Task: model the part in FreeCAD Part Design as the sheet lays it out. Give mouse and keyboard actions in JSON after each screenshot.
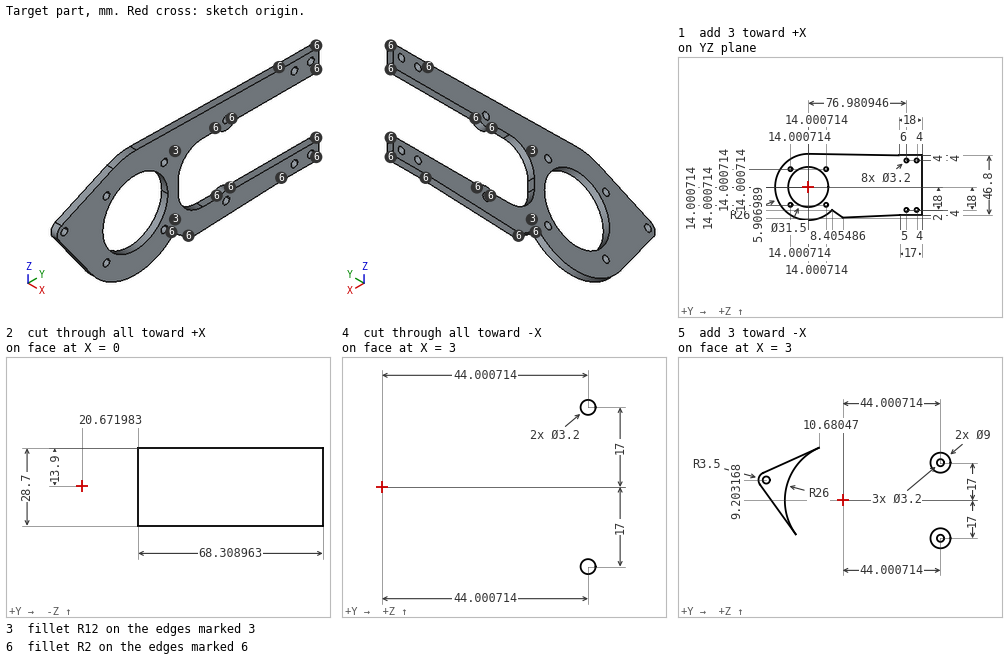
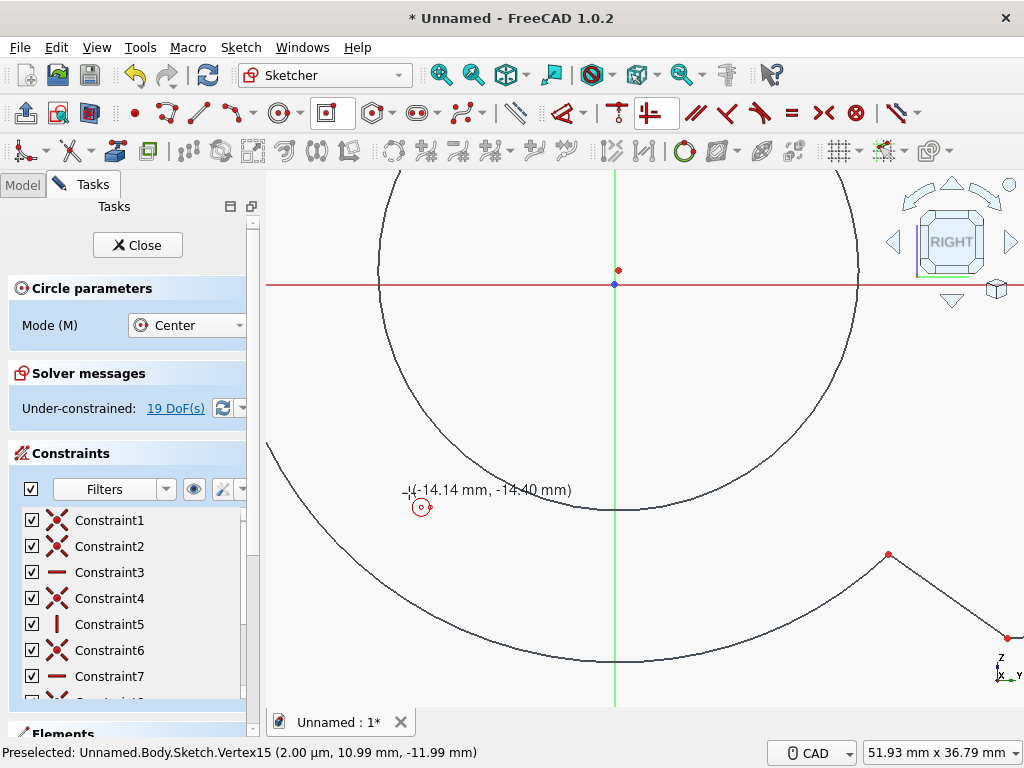
{"action": "scroll", "coordinate": [409, 494], "scroll_direction": "down", "scroll_amount": 7}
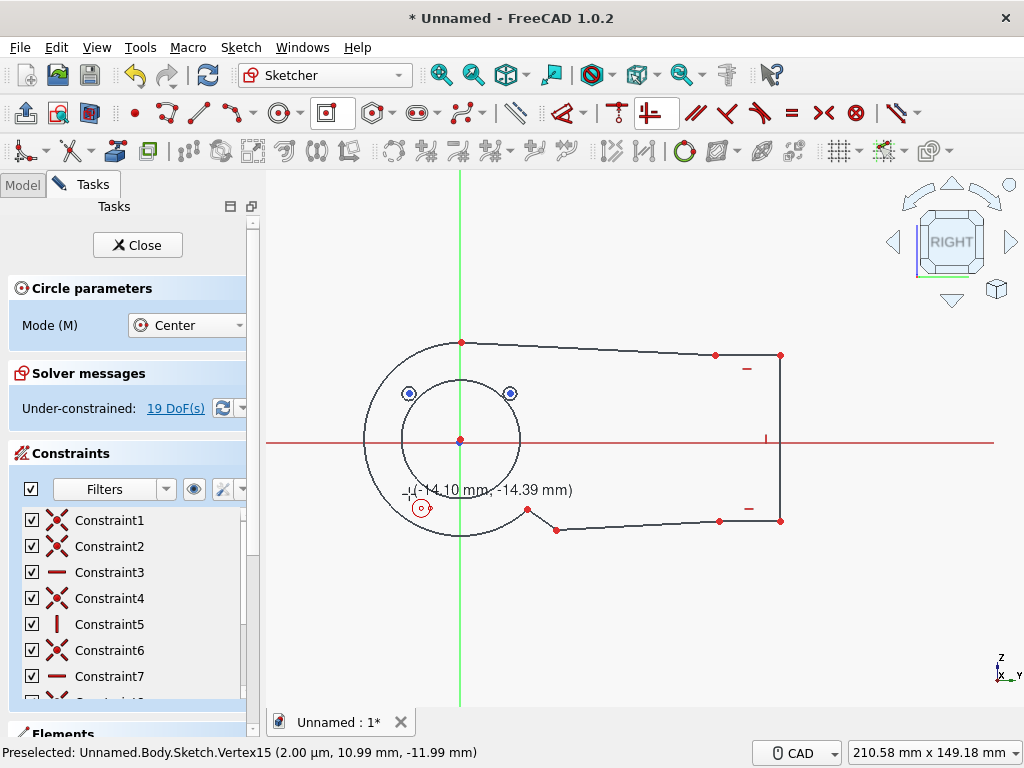
{"action": "left_click", "coordinate": [409, 493]}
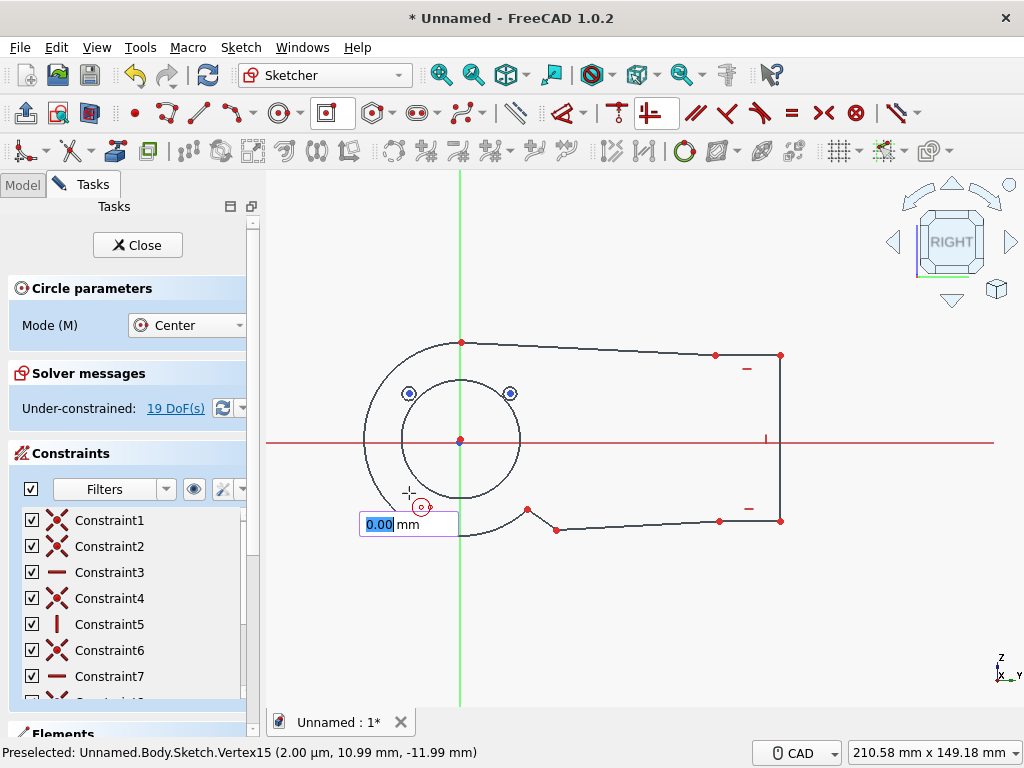
{"action": "scroll", "coordinate": [405, 489], "scroll_direction": "up", "scroll_amount": 6}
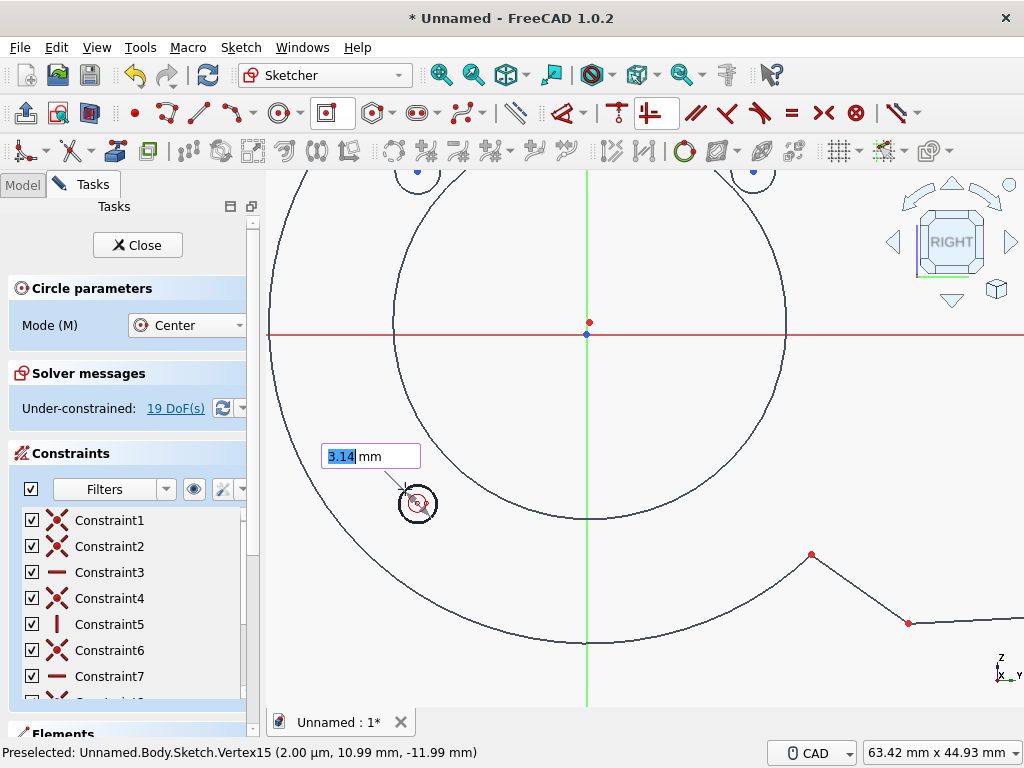
{"action": "left_click", "coordinate": [406, 488]}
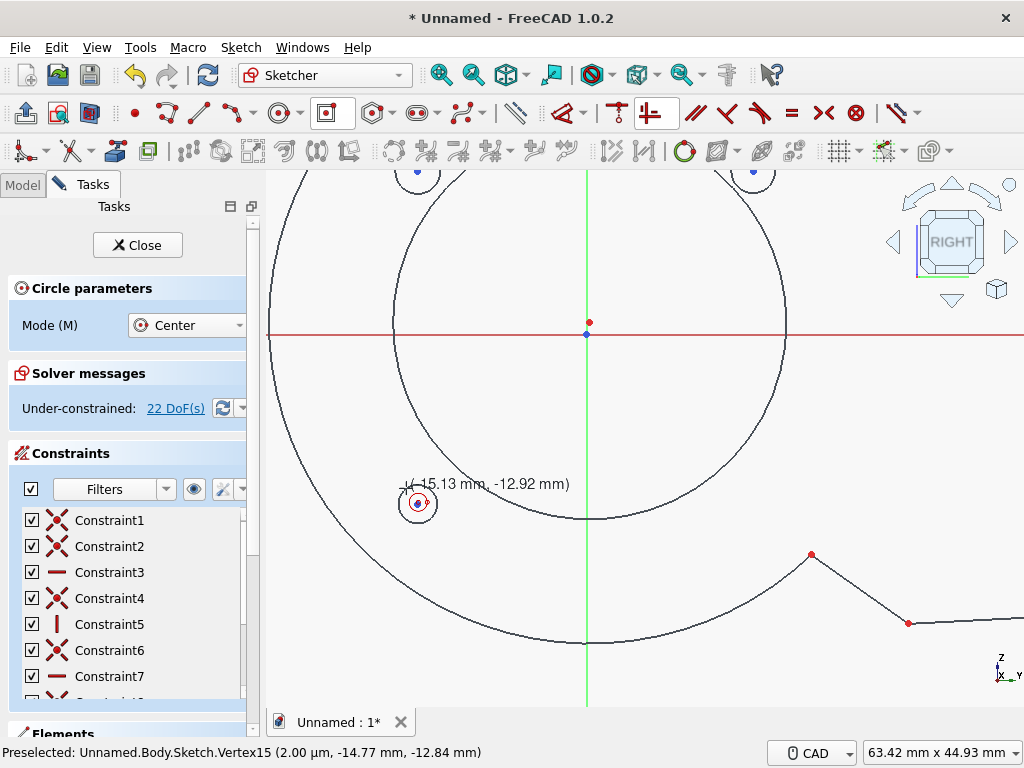
{"action": "scroll", "coordinate": [405, 488], "scroll_direction": "down", "scroll_amount": 6}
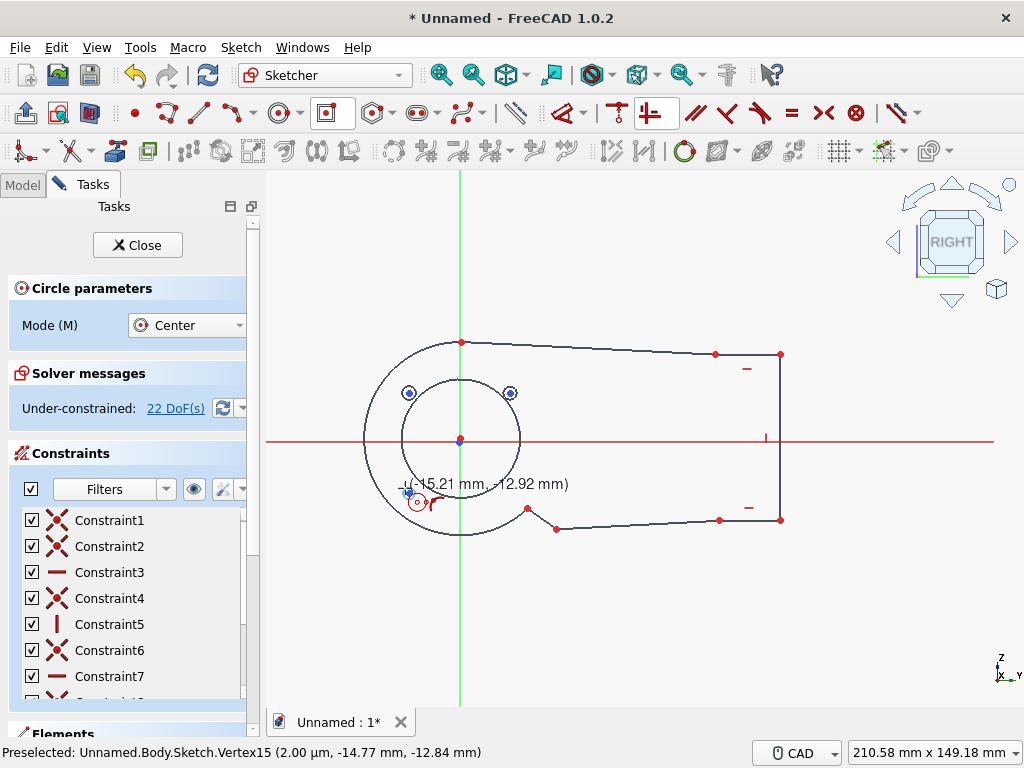
{"action": "left_click", "coordinate": [510, 493]}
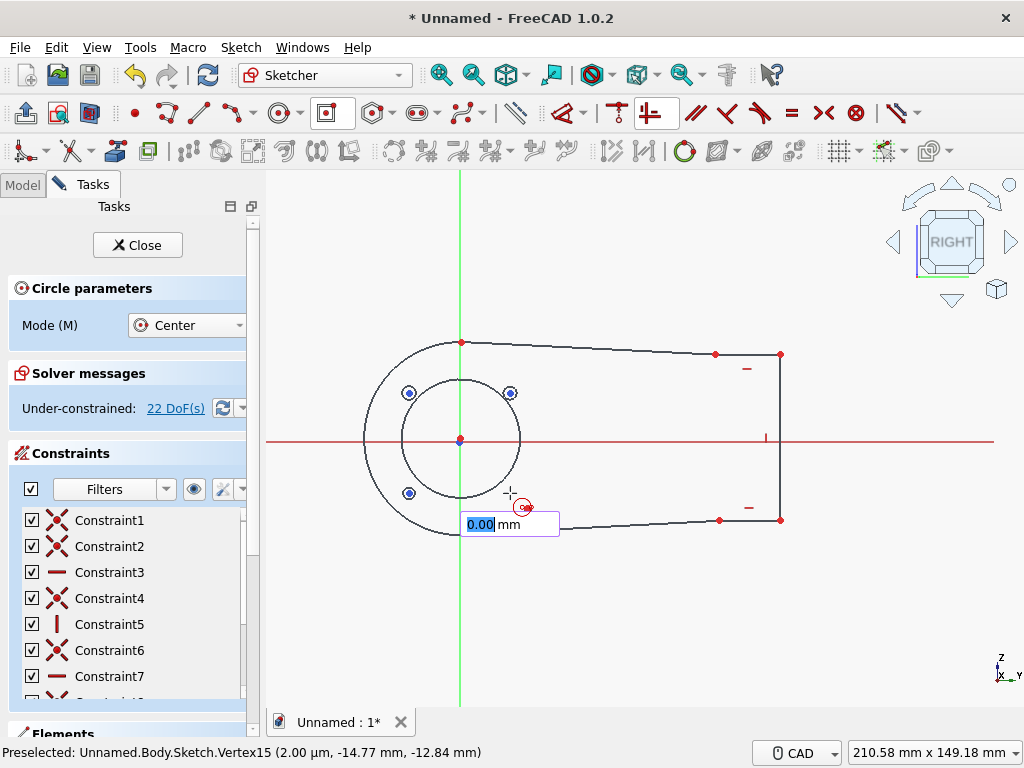
{"action": "scroll", "coordinate": [514, 489], "scroll_direction": "up", "scroll_amount": 6}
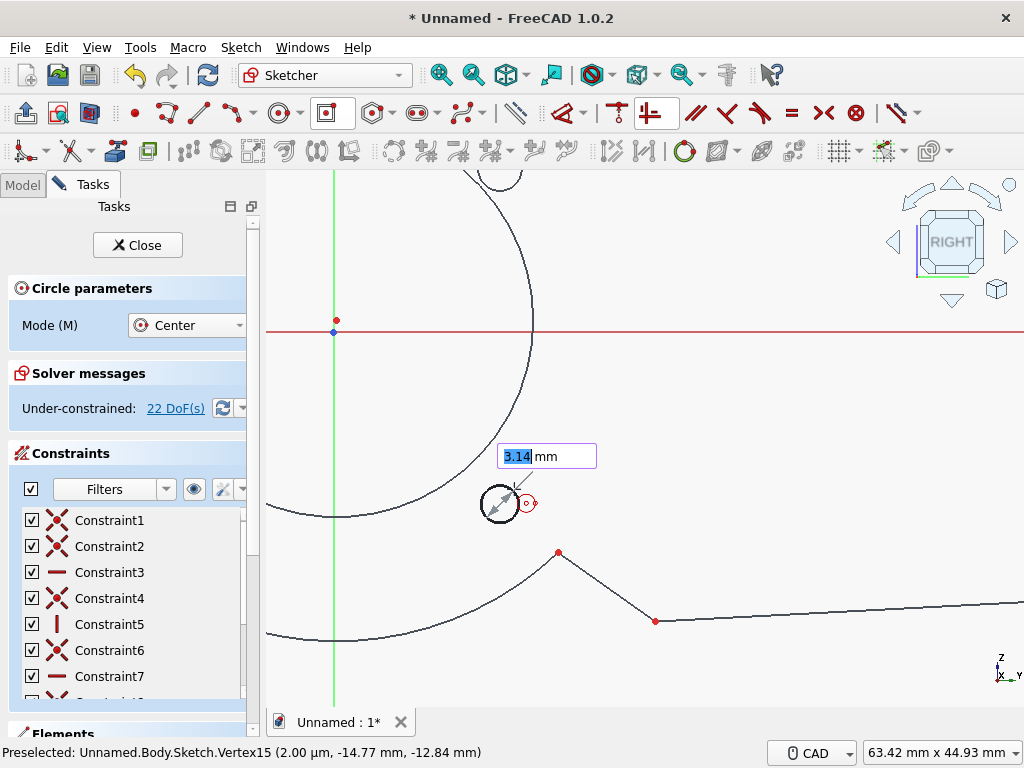
{"action": "left_click", "coordinate": [514, 486]}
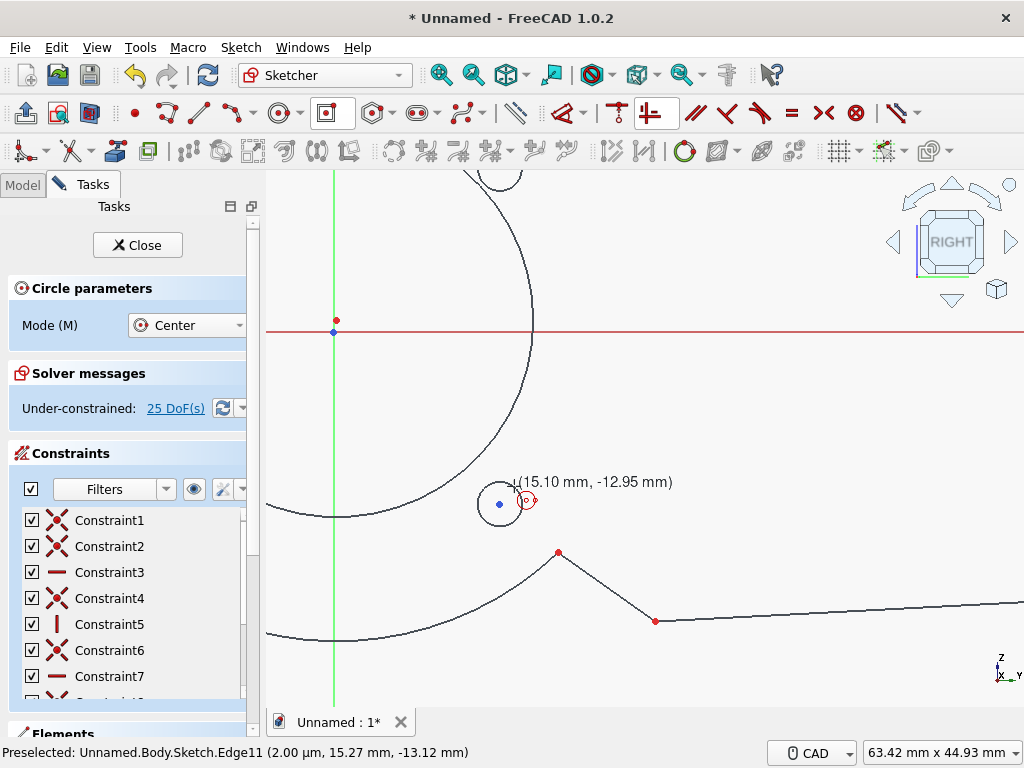
{"action": "scroll", "coordinate": [514, 489], "scroll_direction": "down", "scroll_amount": 6}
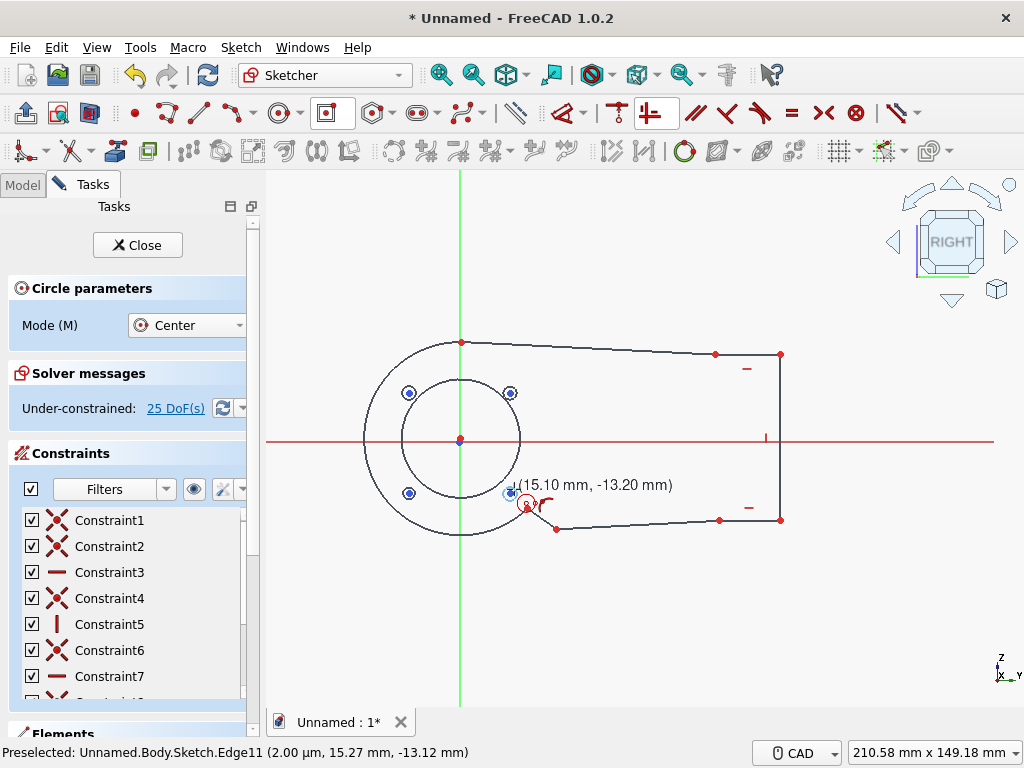
{"action": "scroll", "coordinate": [737, 367], "scroll_direction": "up", "scroll_amount": 7}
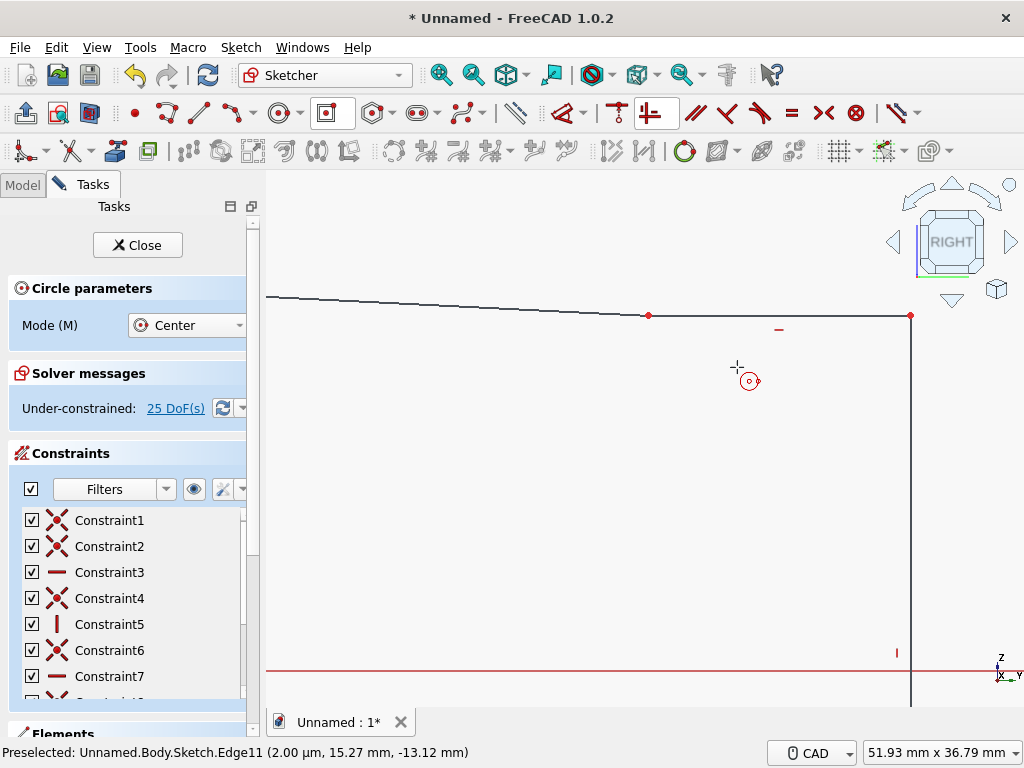
{"action": "scroll", "coordinate": [737, 367], "scroll_direction": "down", "scroll_amount": 7}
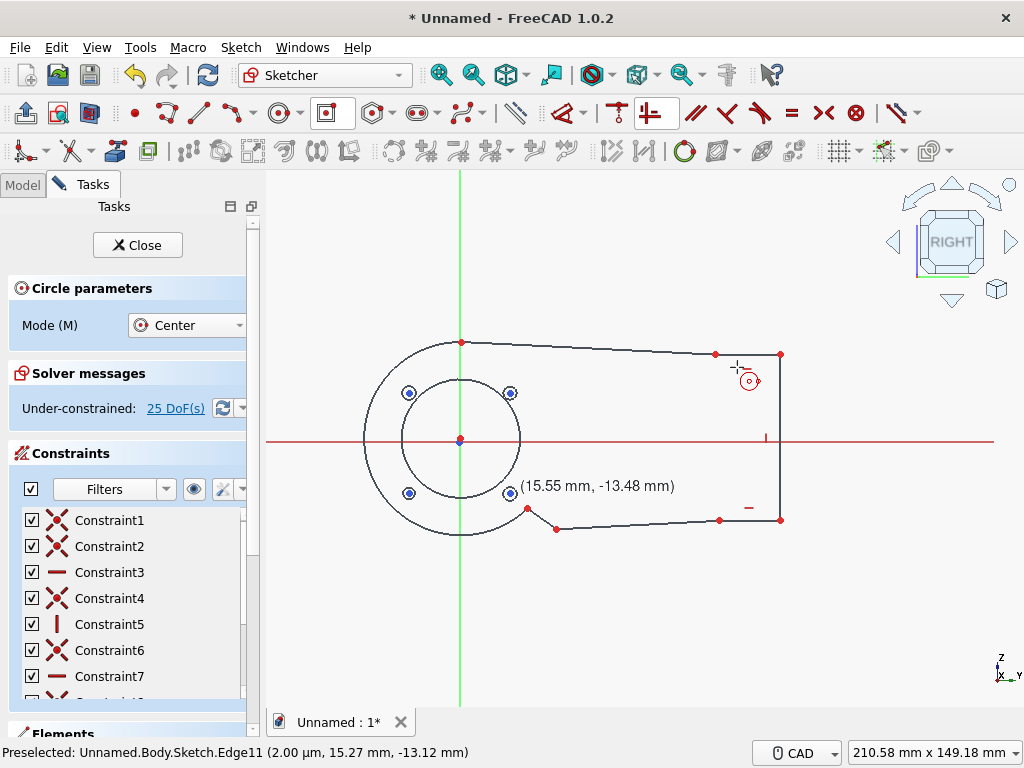
{"action": "left_click", "coordinate": [737, 367]}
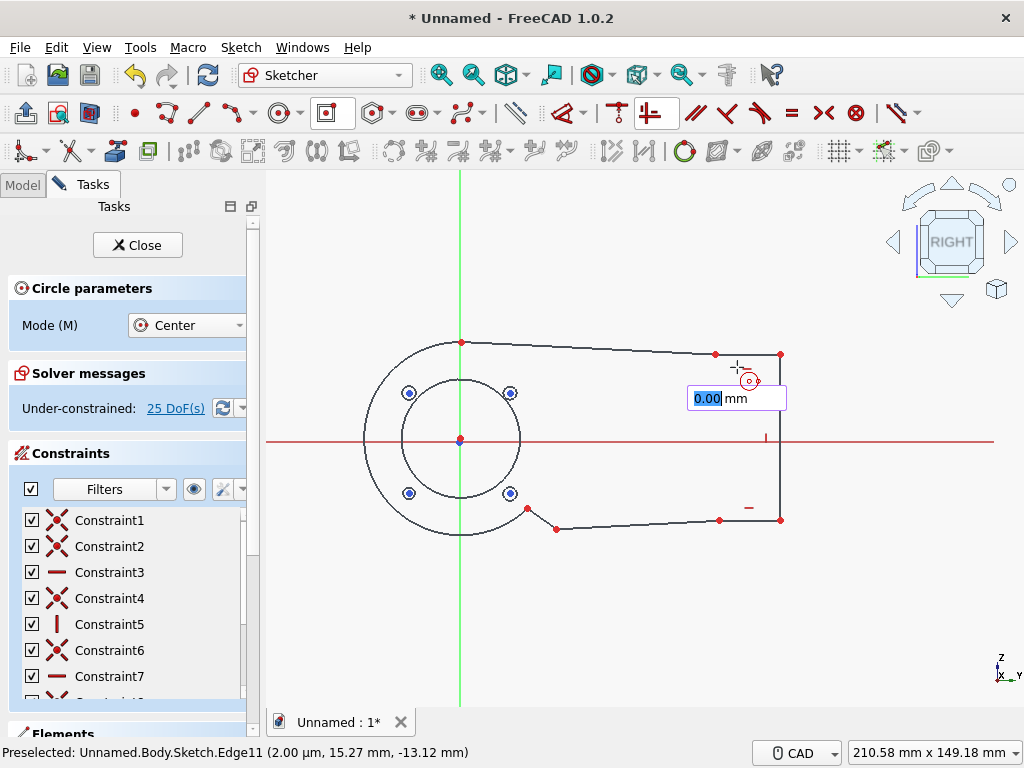
{"action": "scroll", "coordinate": [741, 371], "scroll_direction": "up", "scroll_amount": 6}